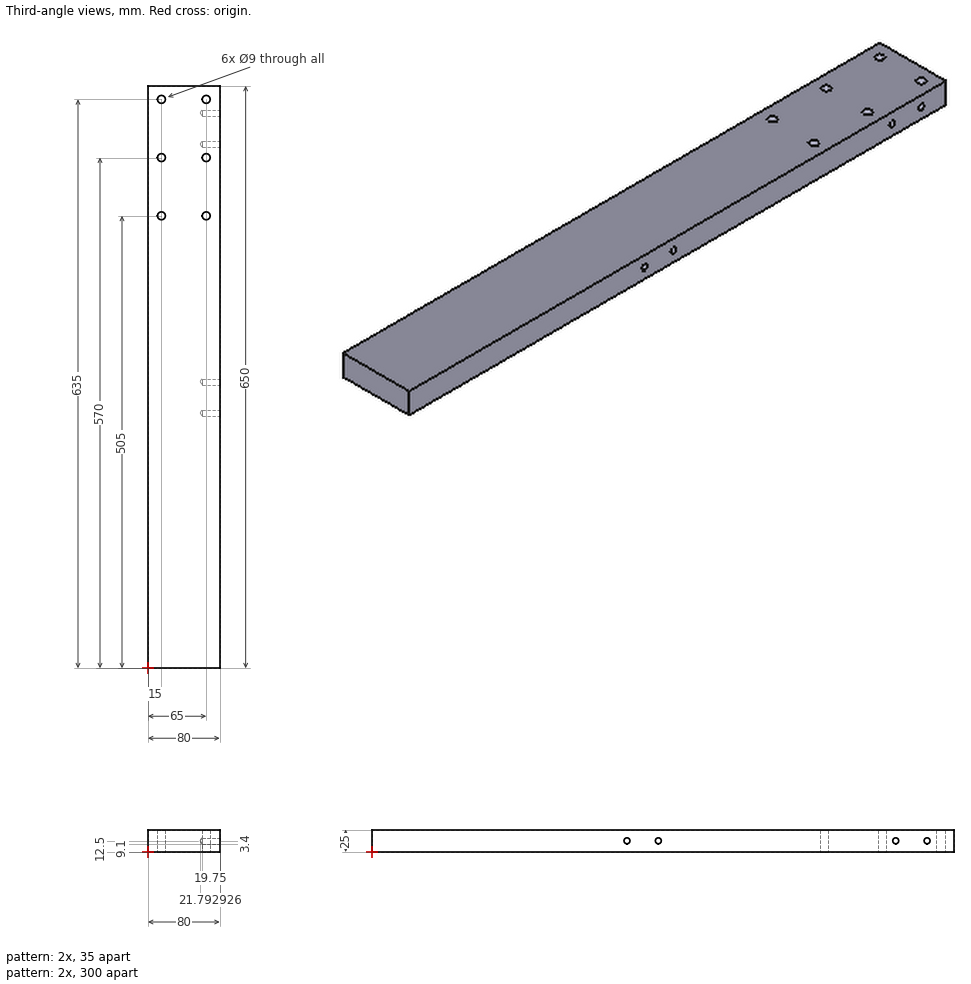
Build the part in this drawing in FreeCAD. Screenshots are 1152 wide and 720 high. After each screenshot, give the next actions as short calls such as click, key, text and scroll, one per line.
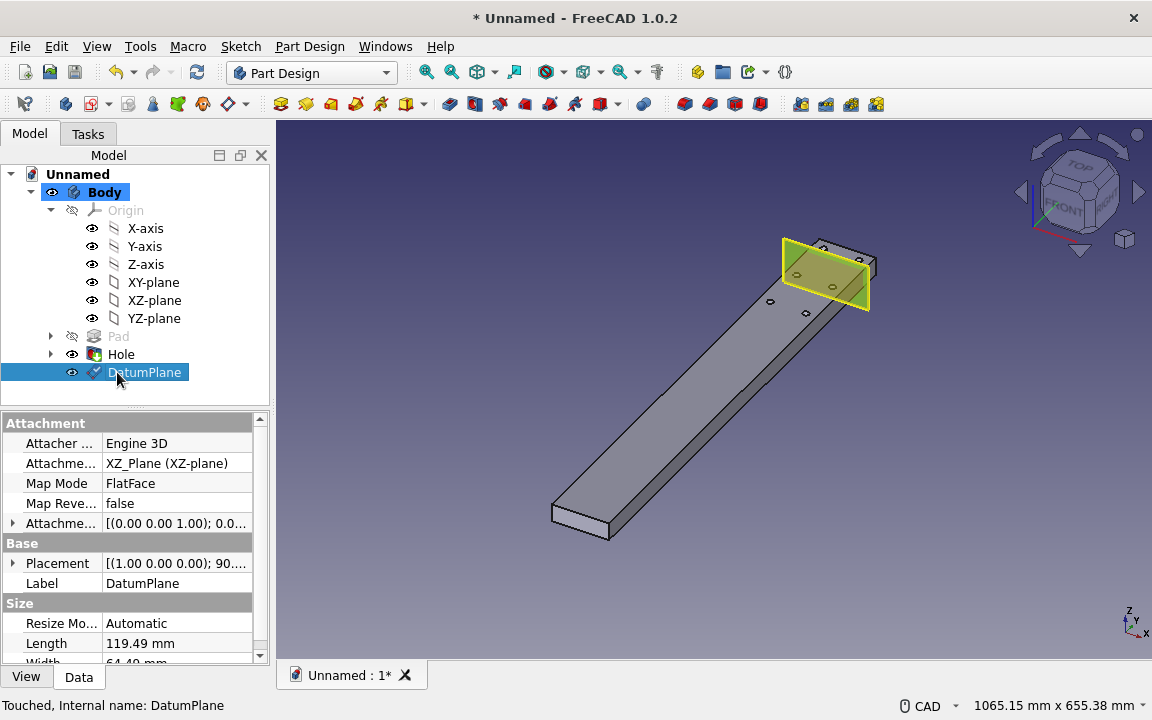
click(90, 104)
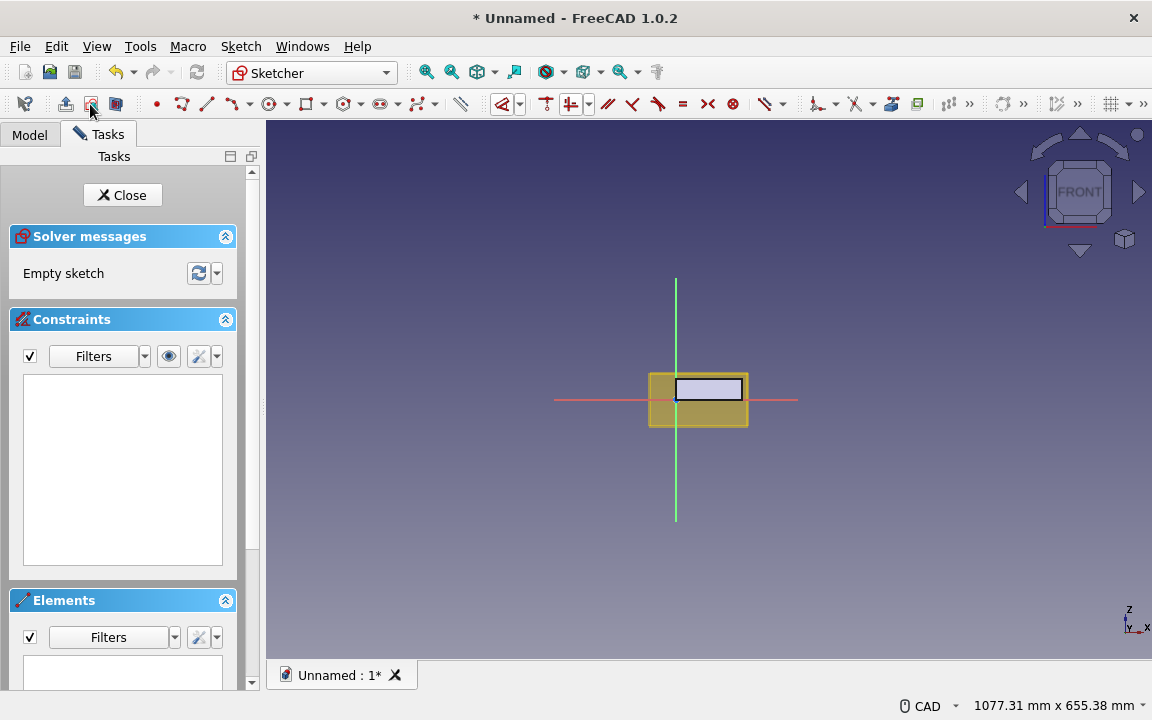
key(q)
key(s)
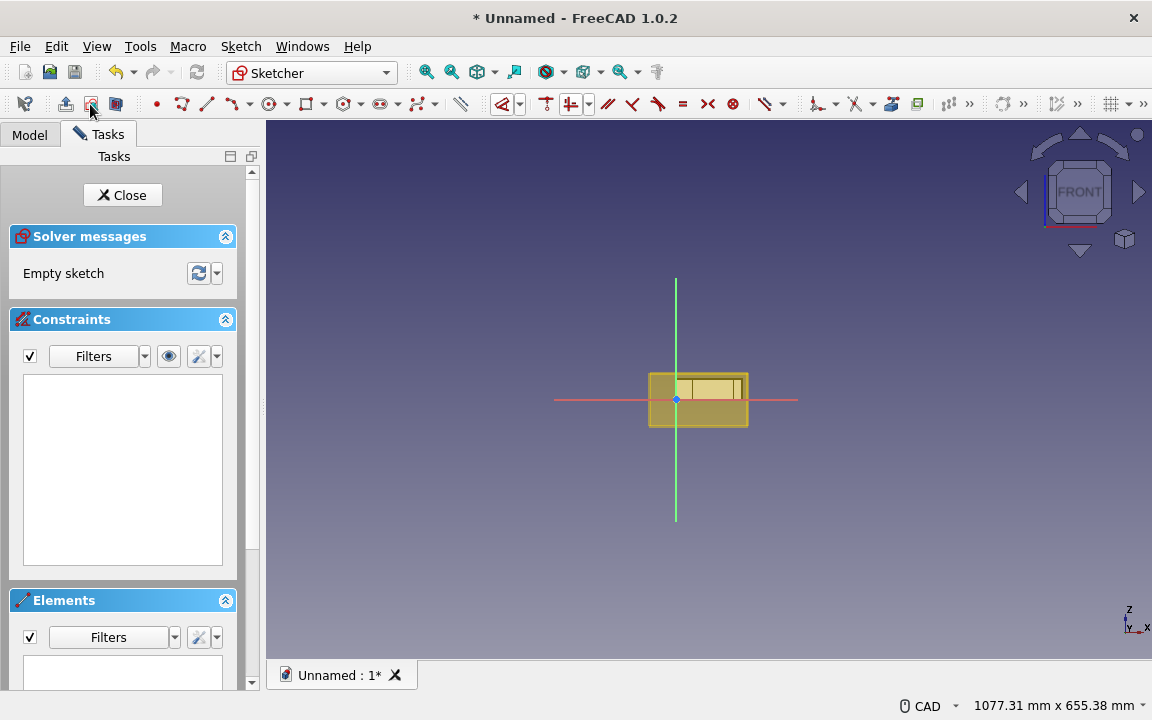
scroll(734, 391, up, 15)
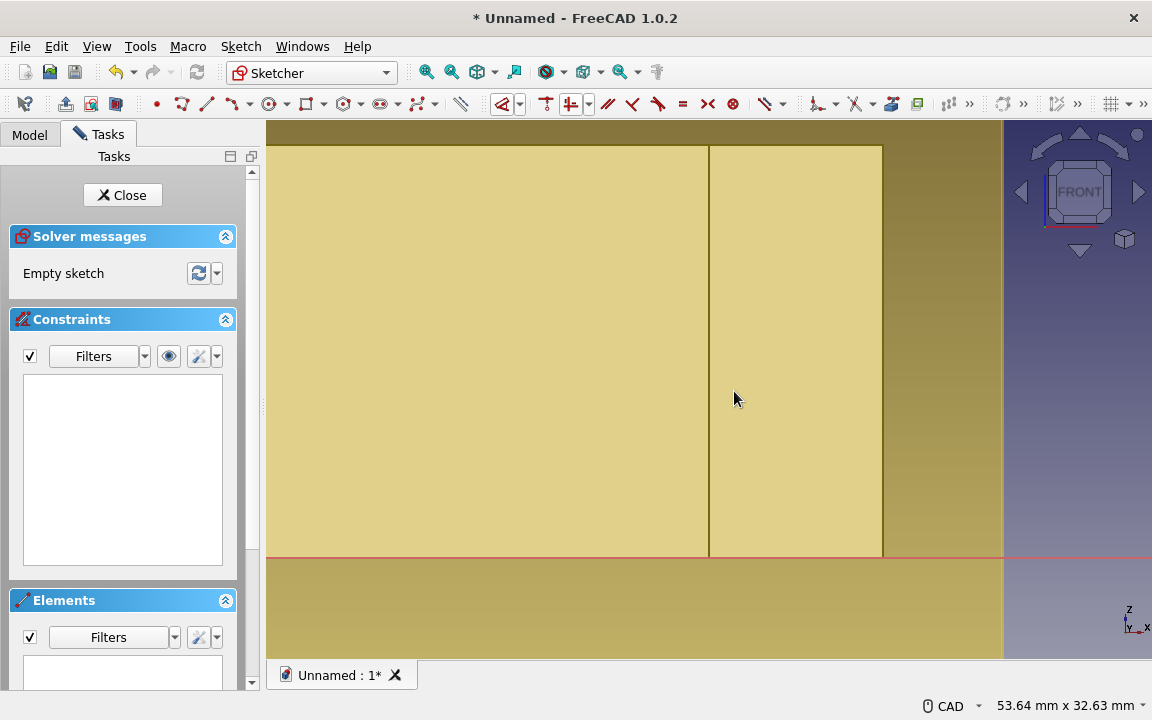
key(g)
key(m)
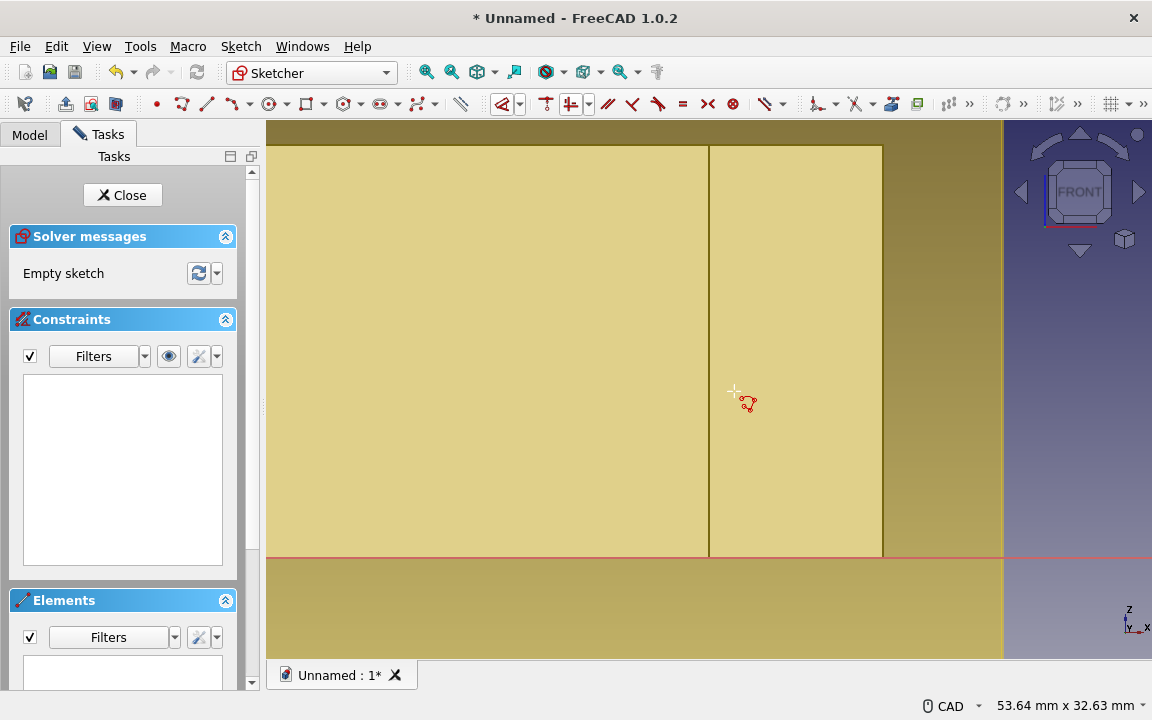
click(523, 351)
click(883, 351)
click(883, 407)
click(556, 407)
click(523, 352)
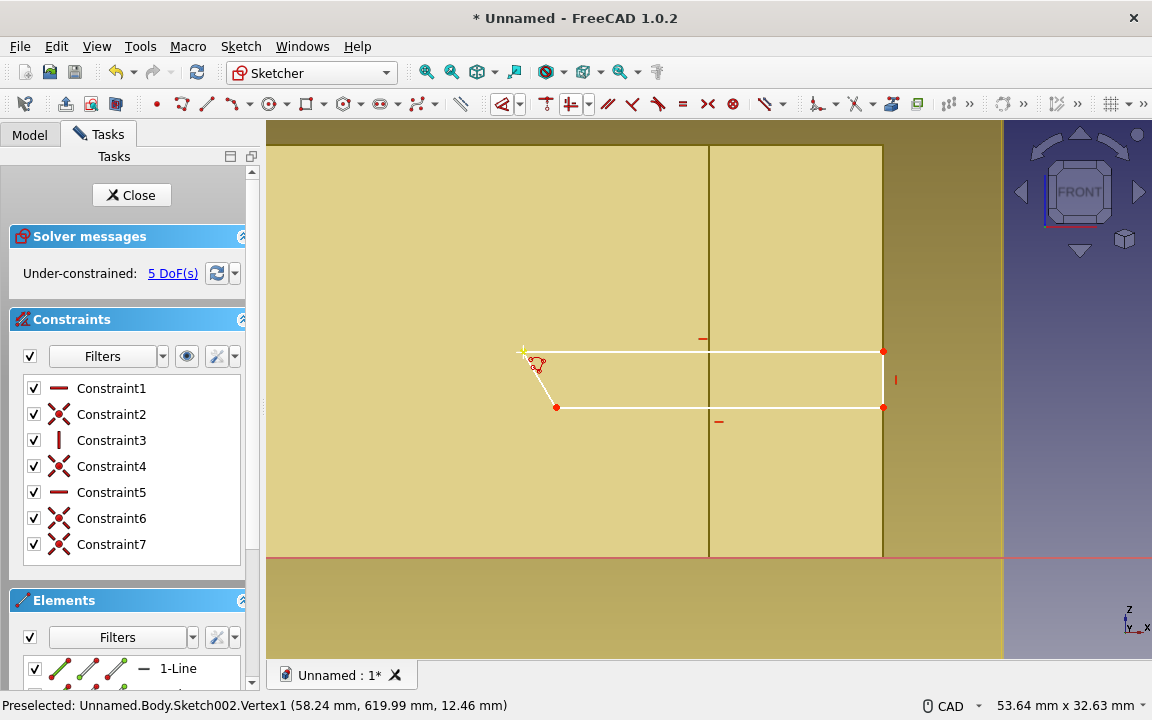
key(g)
key(l)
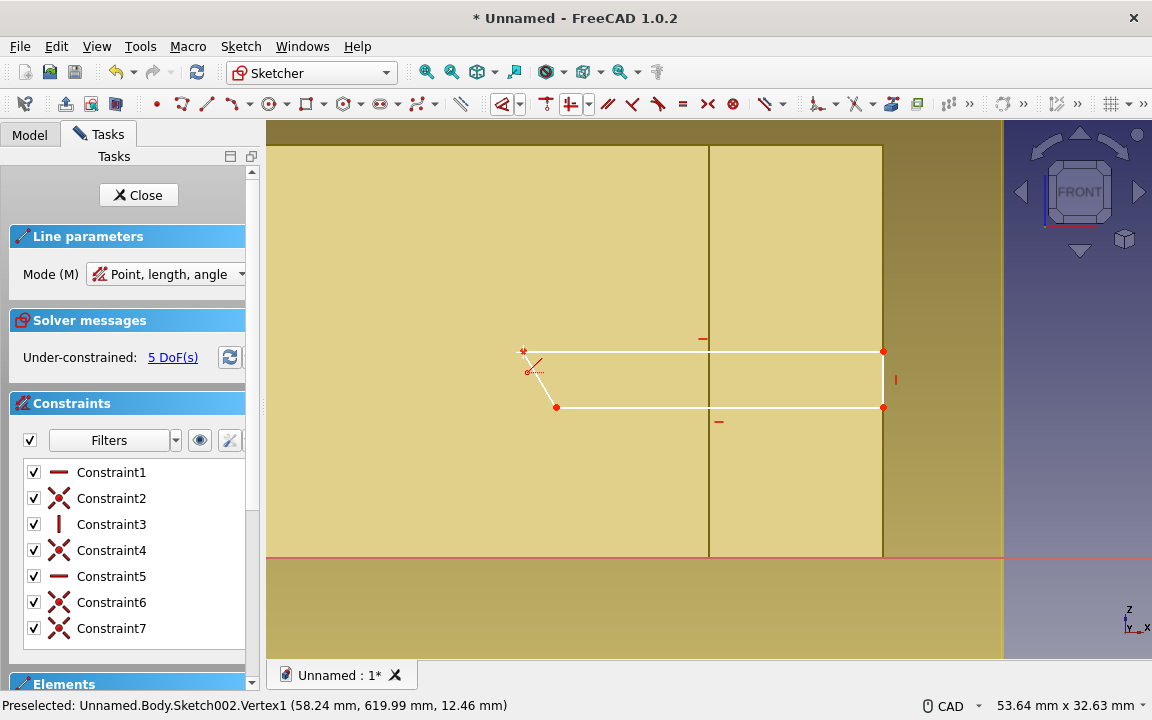
click(487, 351)
click(379, 351)
key(Escape)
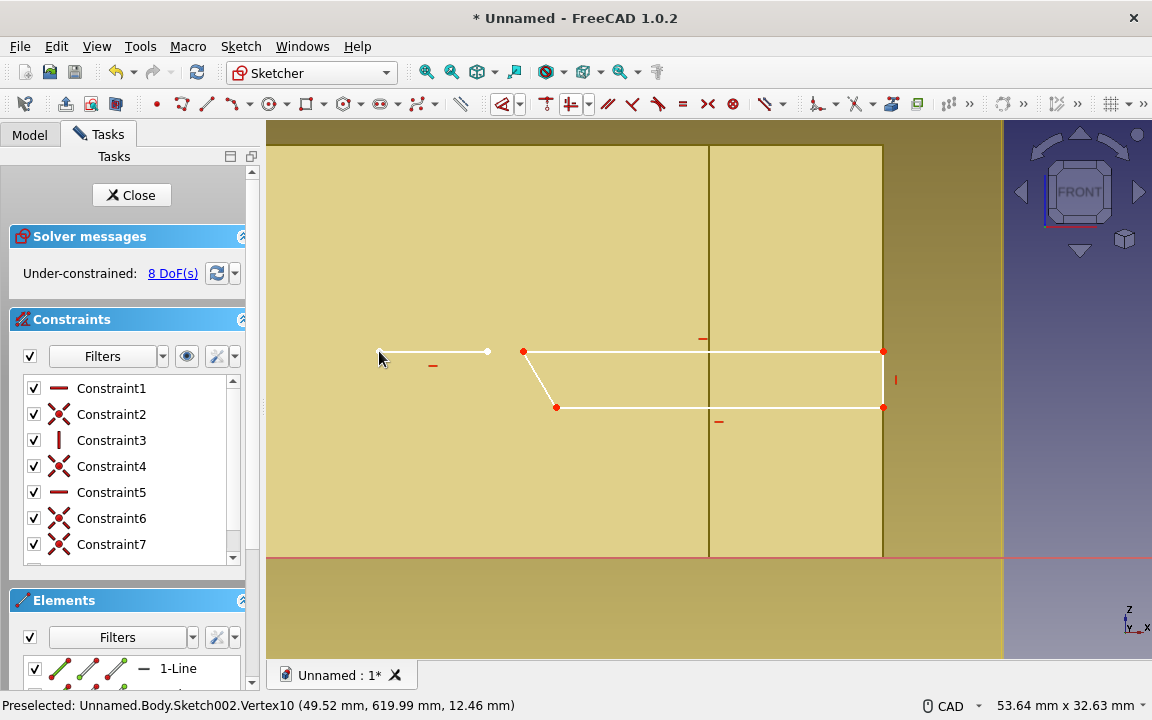
click(455, 352)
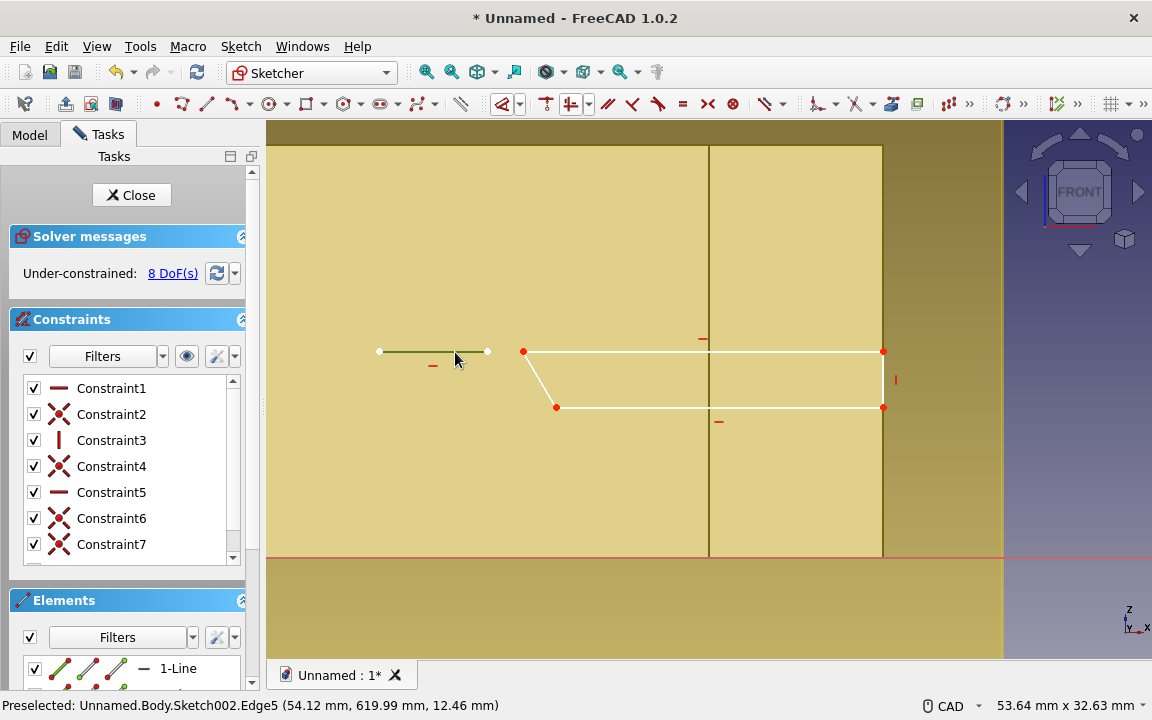
click(461, 104)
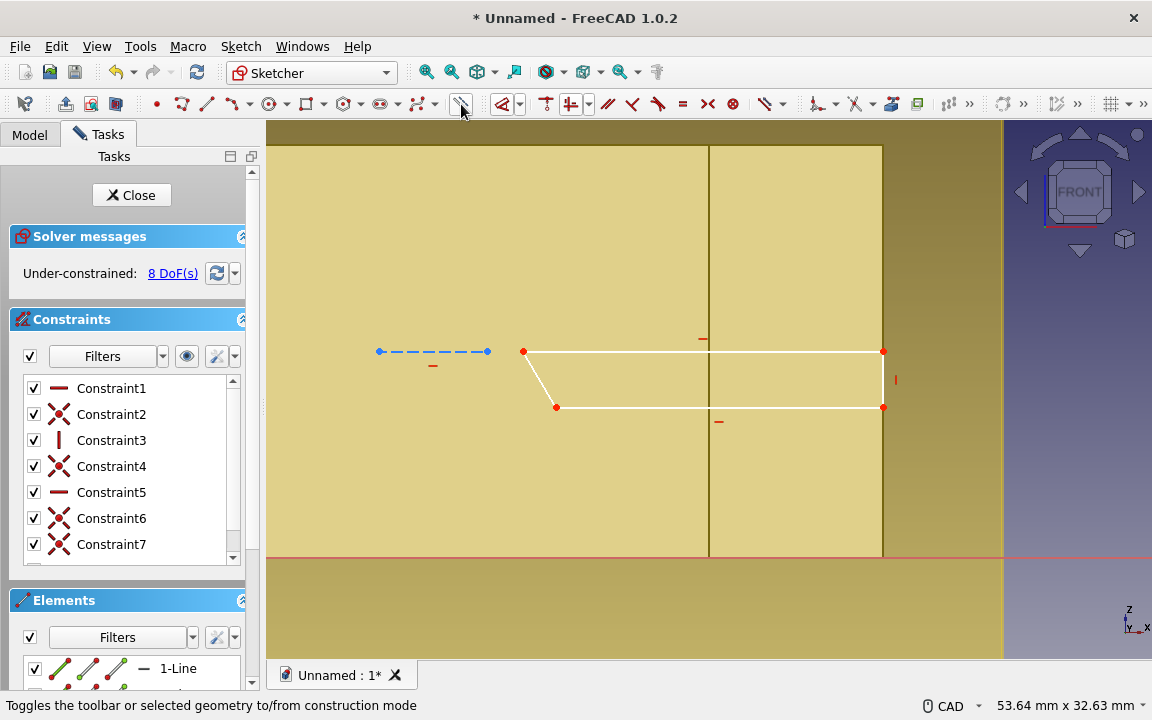
key(d)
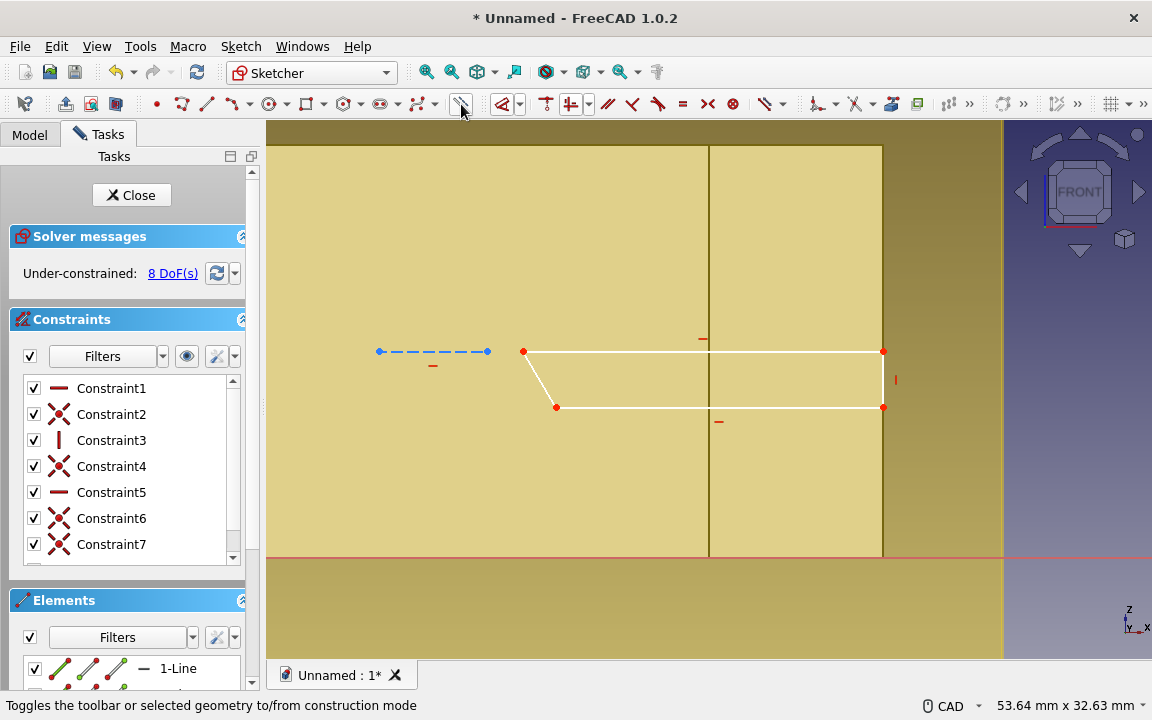
click(883, 369)
click(917, 380)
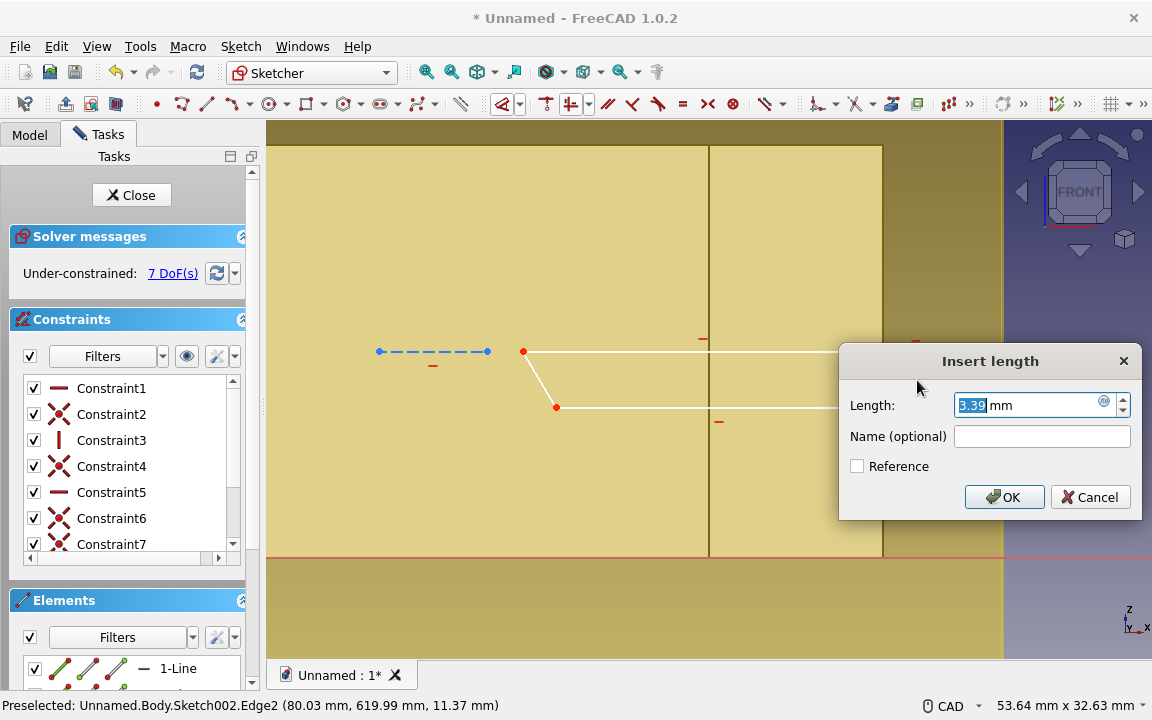
text(3.4)
key(Return)